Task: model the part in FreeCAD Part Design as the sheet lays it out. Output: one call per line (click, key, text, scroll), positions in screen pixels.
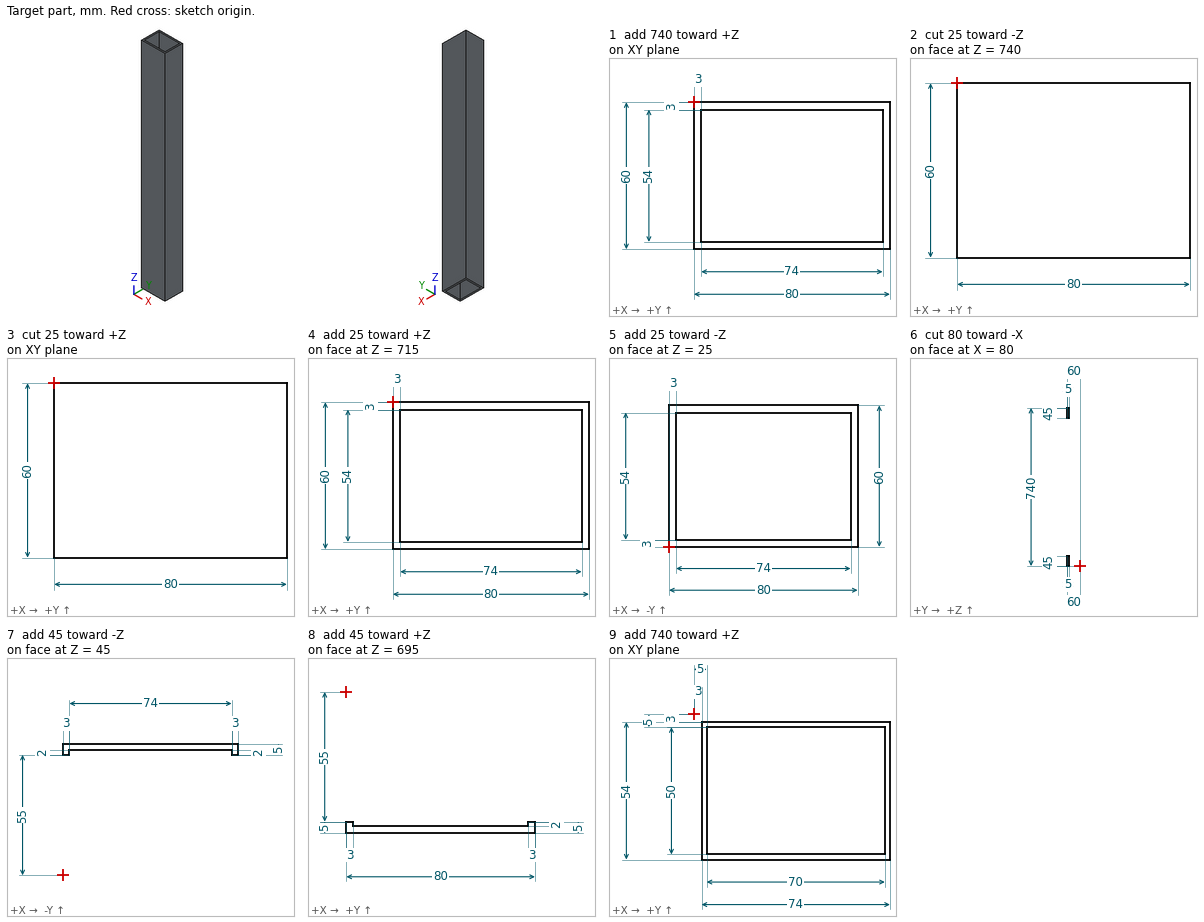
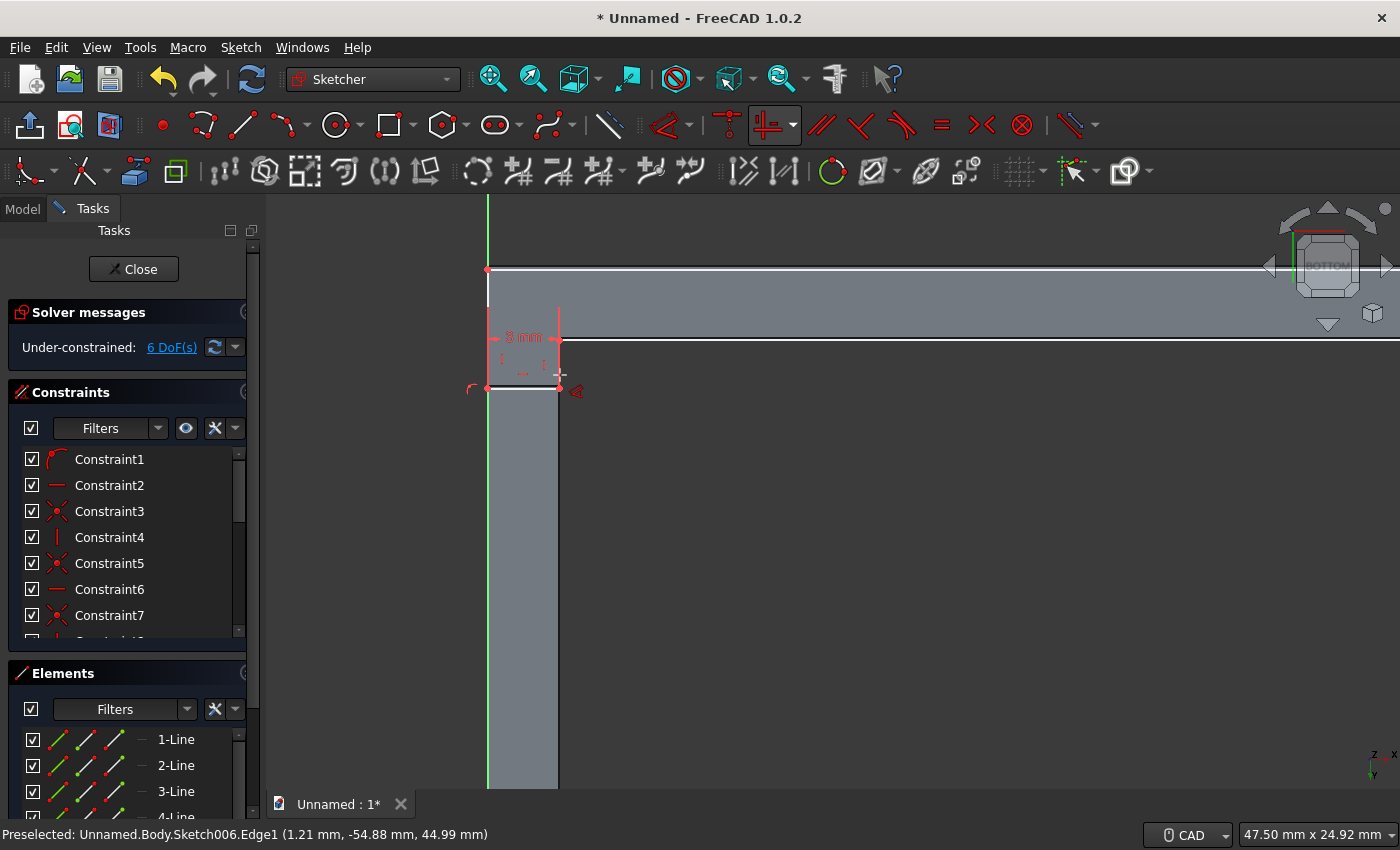
click(559, 374)
click(525, 365)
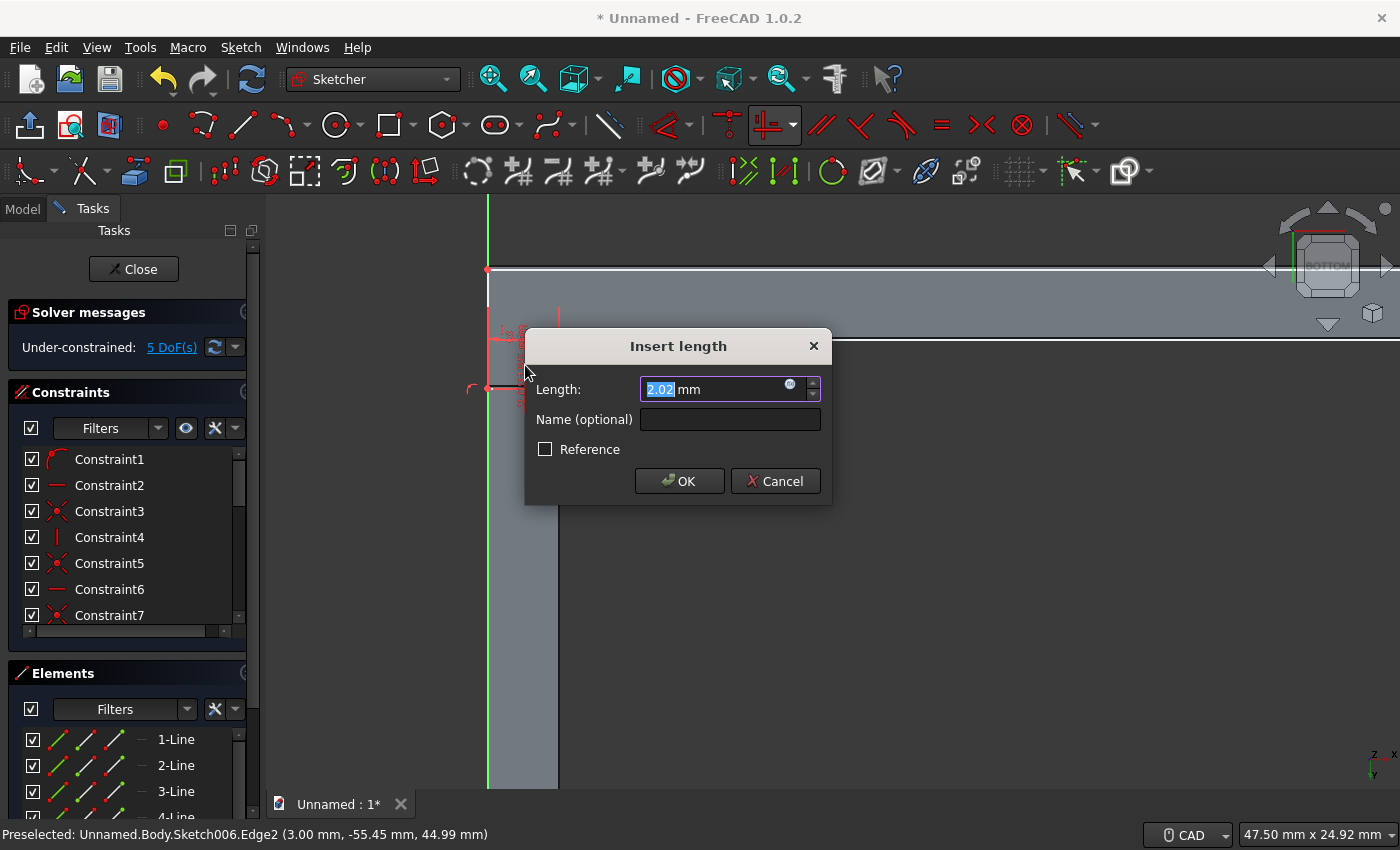
text(2)
key(Return)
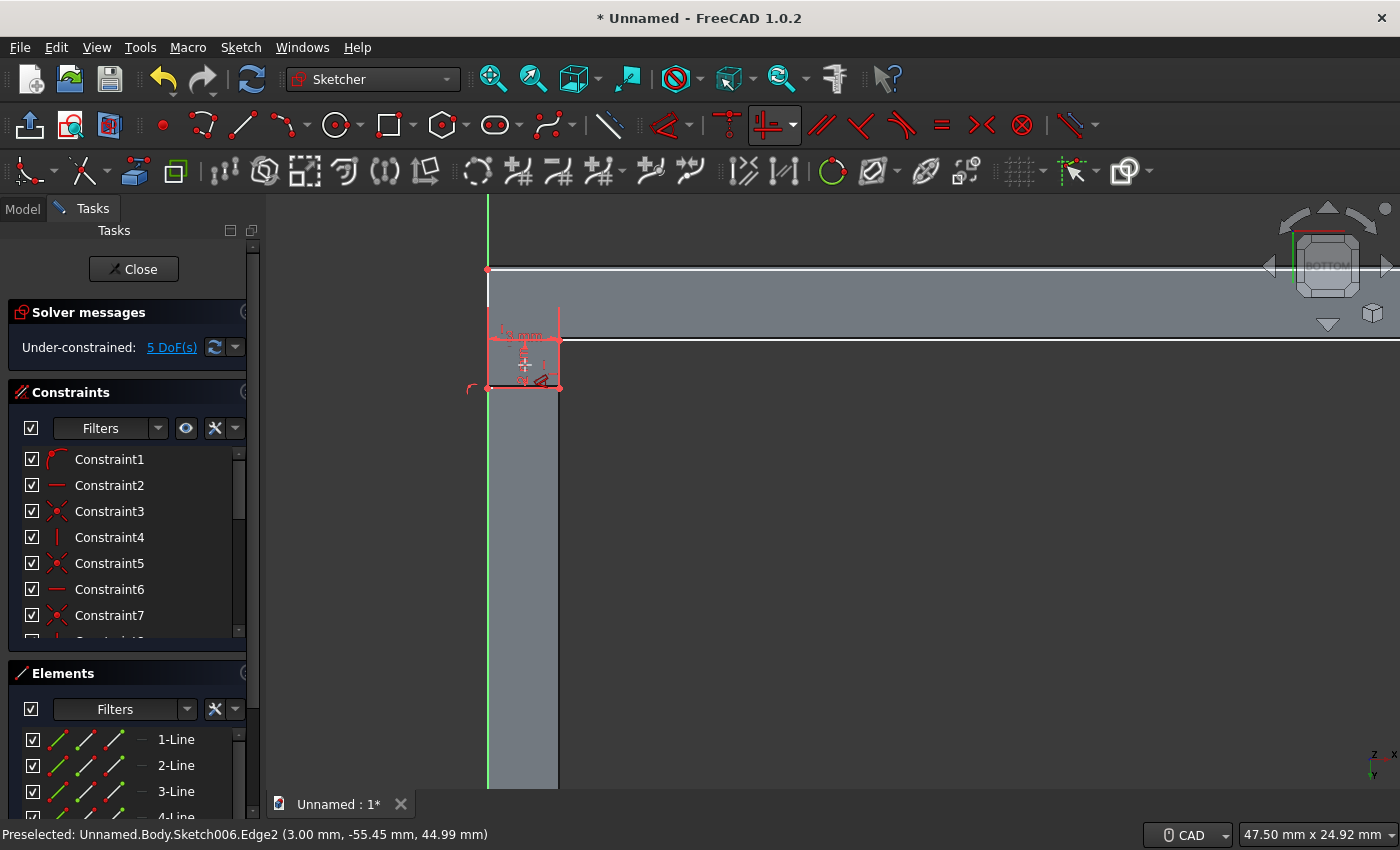
scroll(542, 331, down, 7)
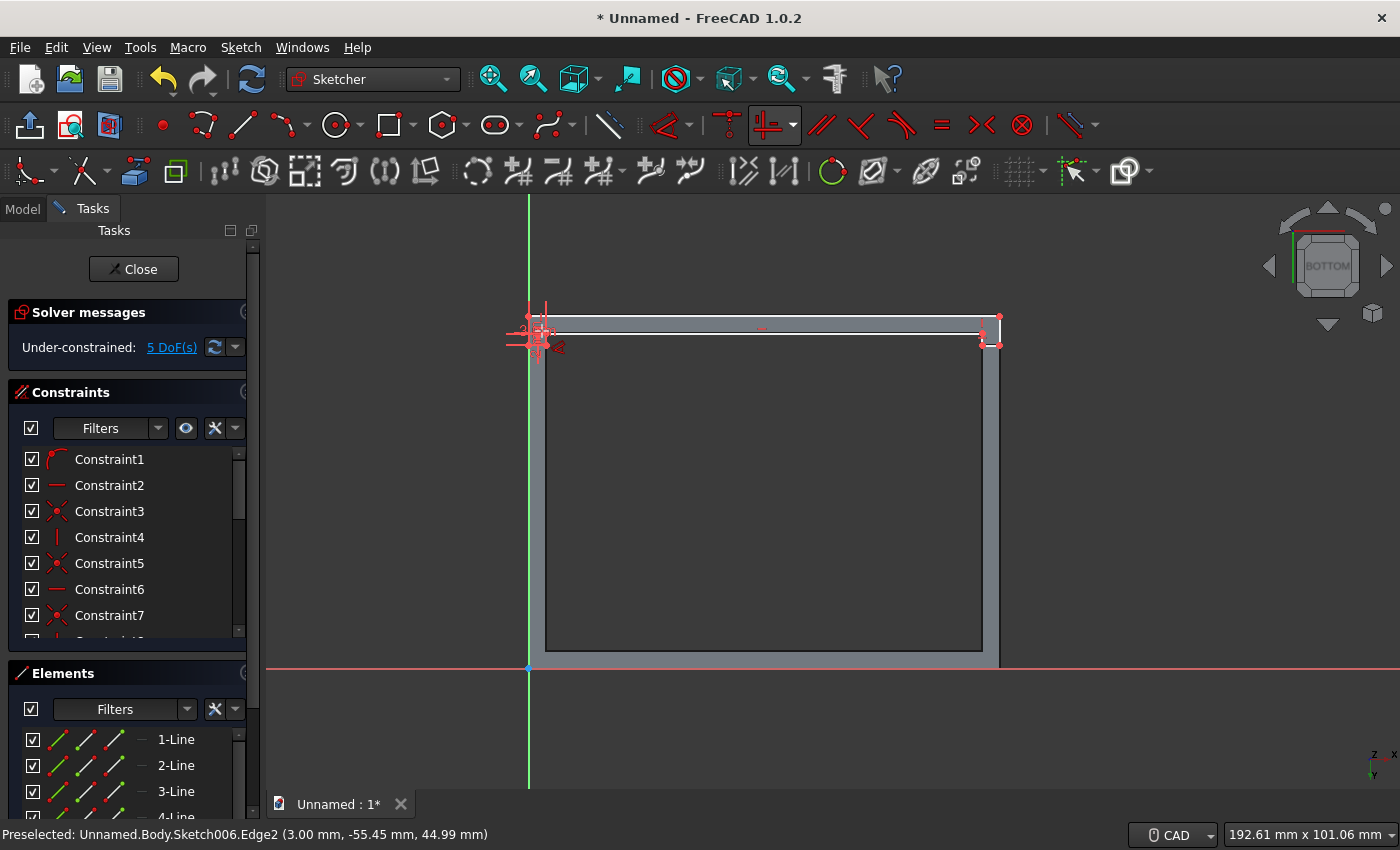
scroll(982, 337, up, 7)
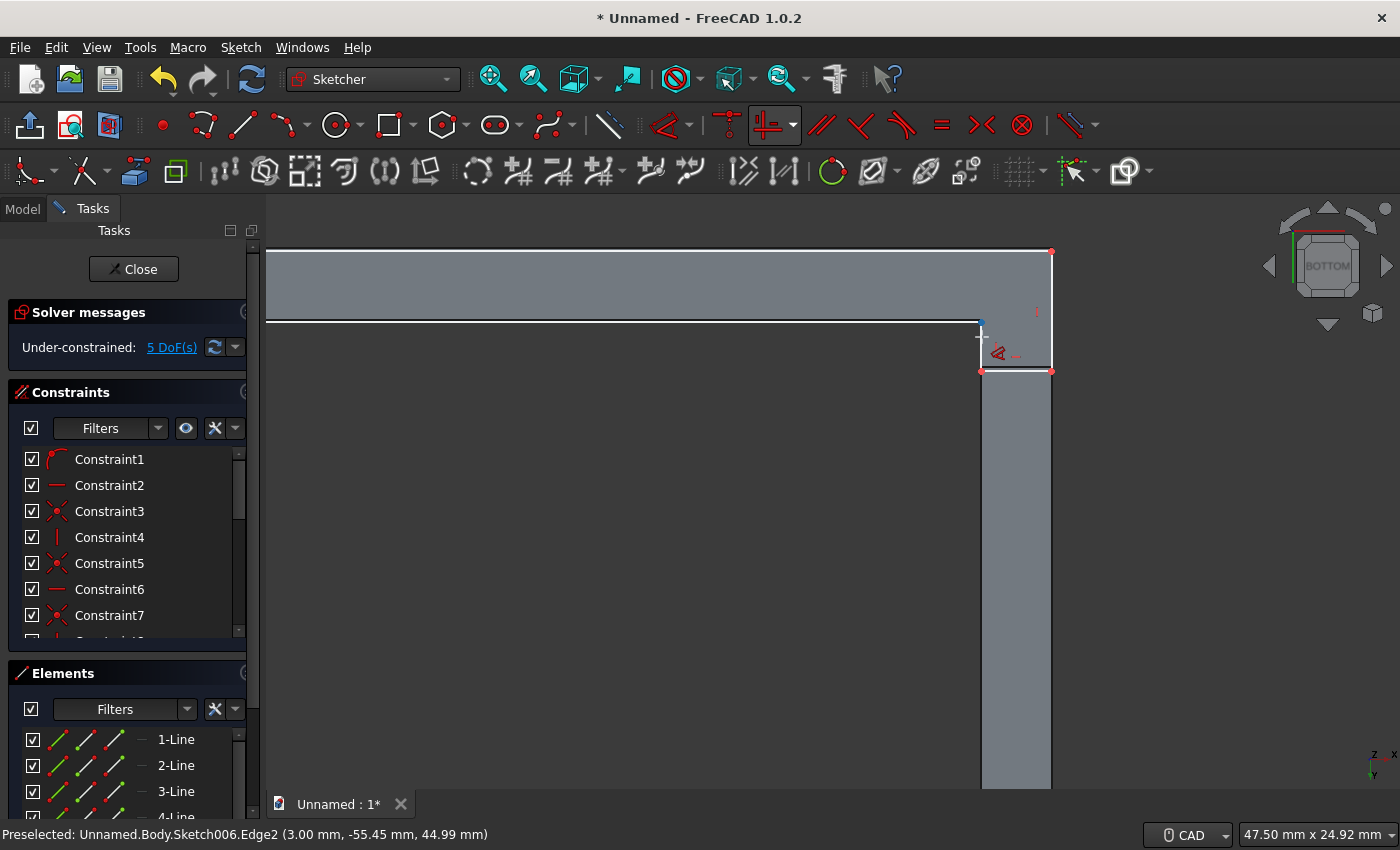
click(981, 337)
click(1015, 347)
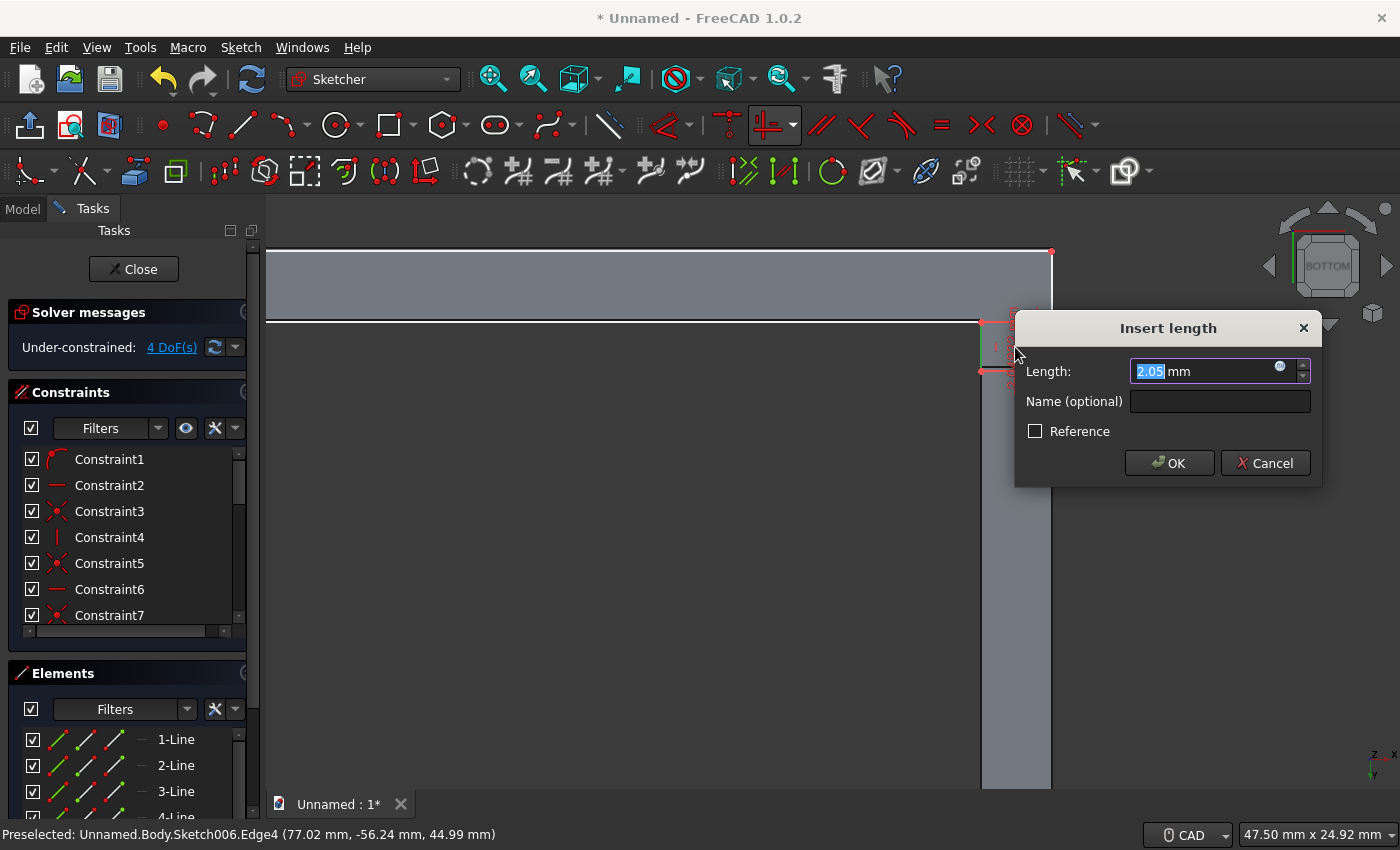
text(2)
key(Return)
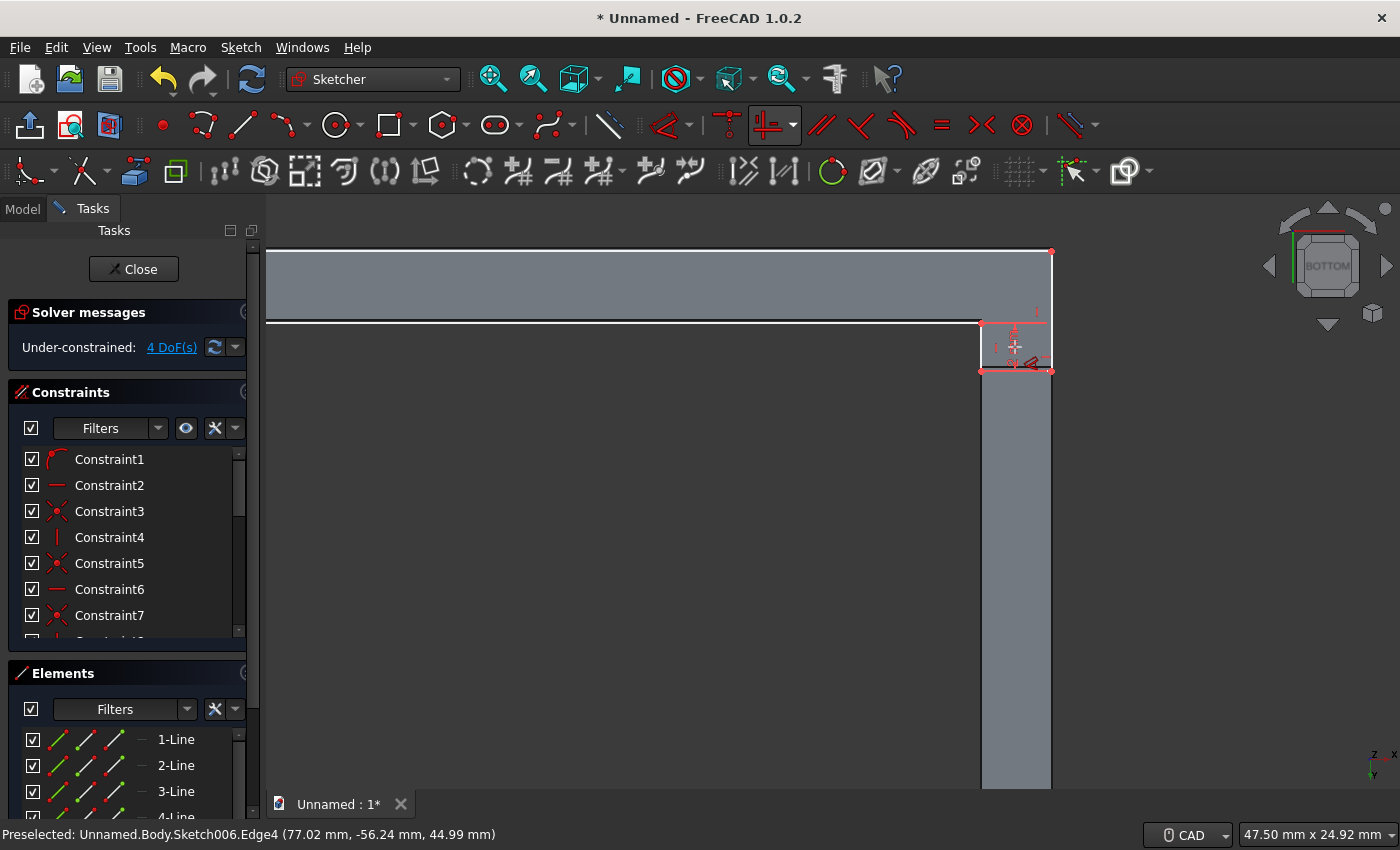
click(1002, 371)
click(1017, 405)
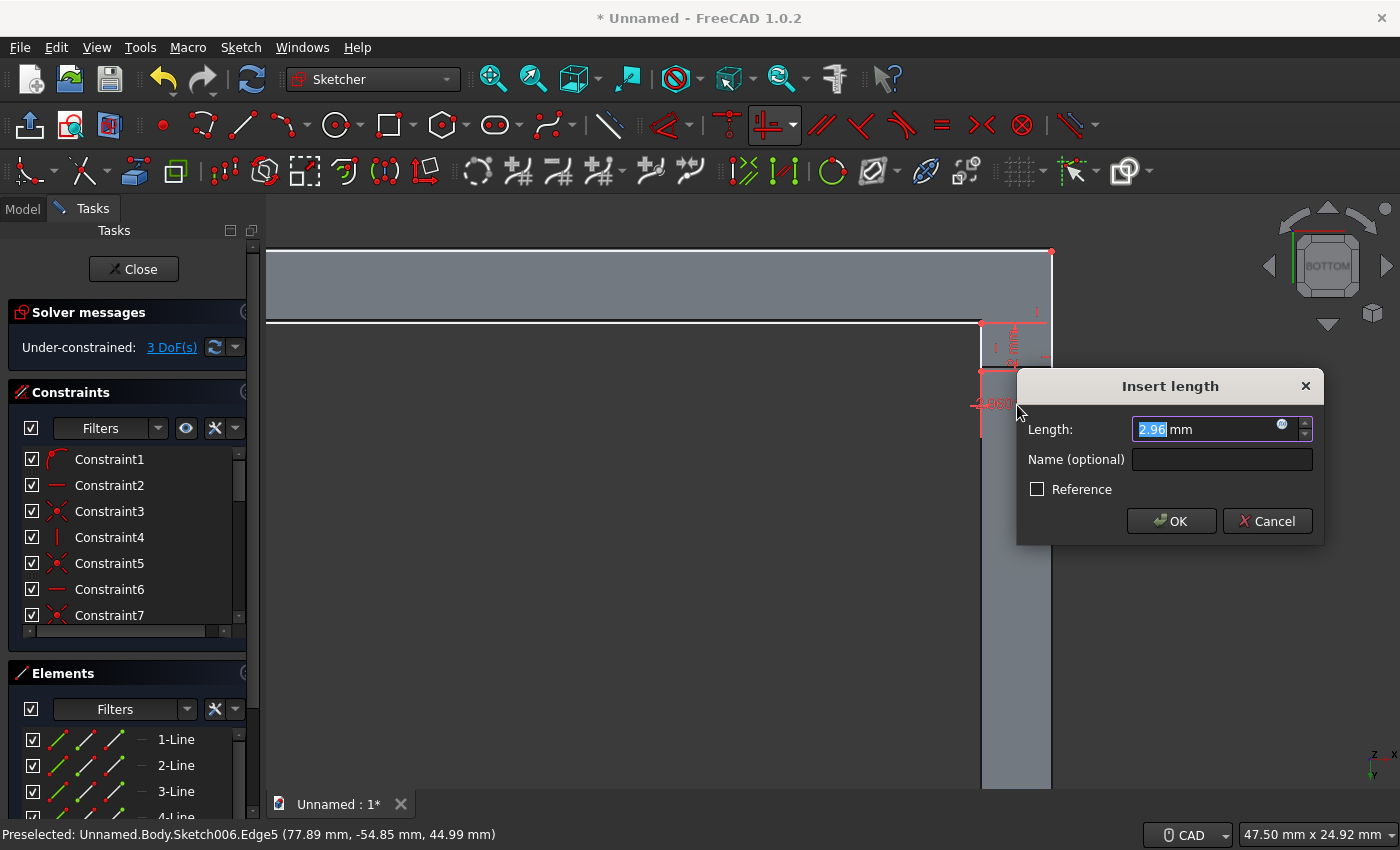
text(3)
key(Return)